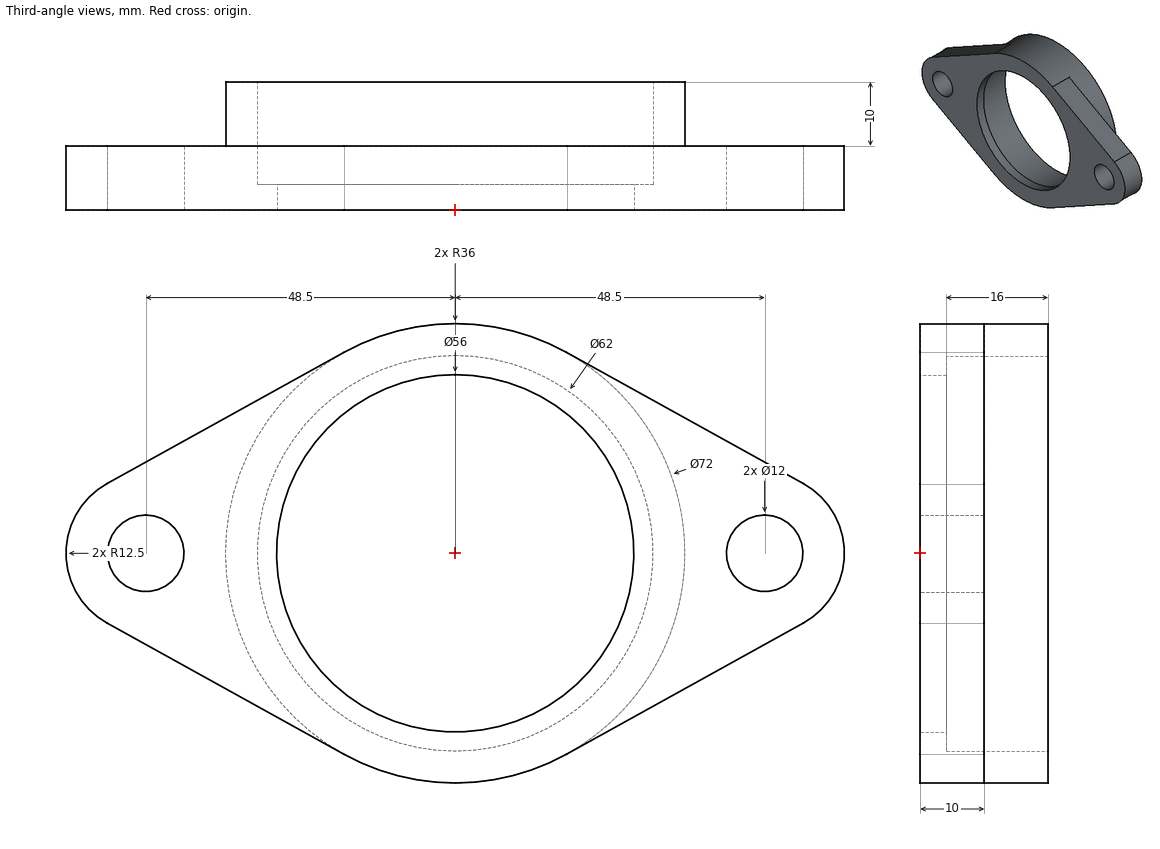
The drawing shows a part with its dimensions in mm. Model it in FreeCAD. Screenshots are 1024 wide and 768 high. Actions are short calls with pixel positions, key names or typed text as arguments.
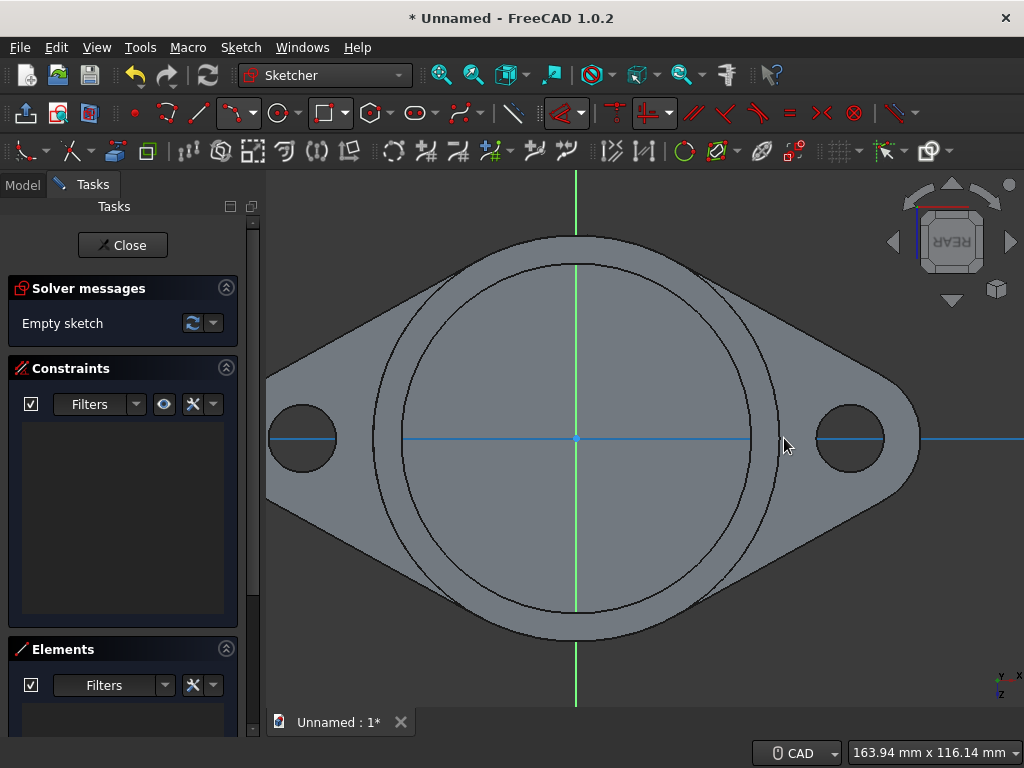
click(278, 114)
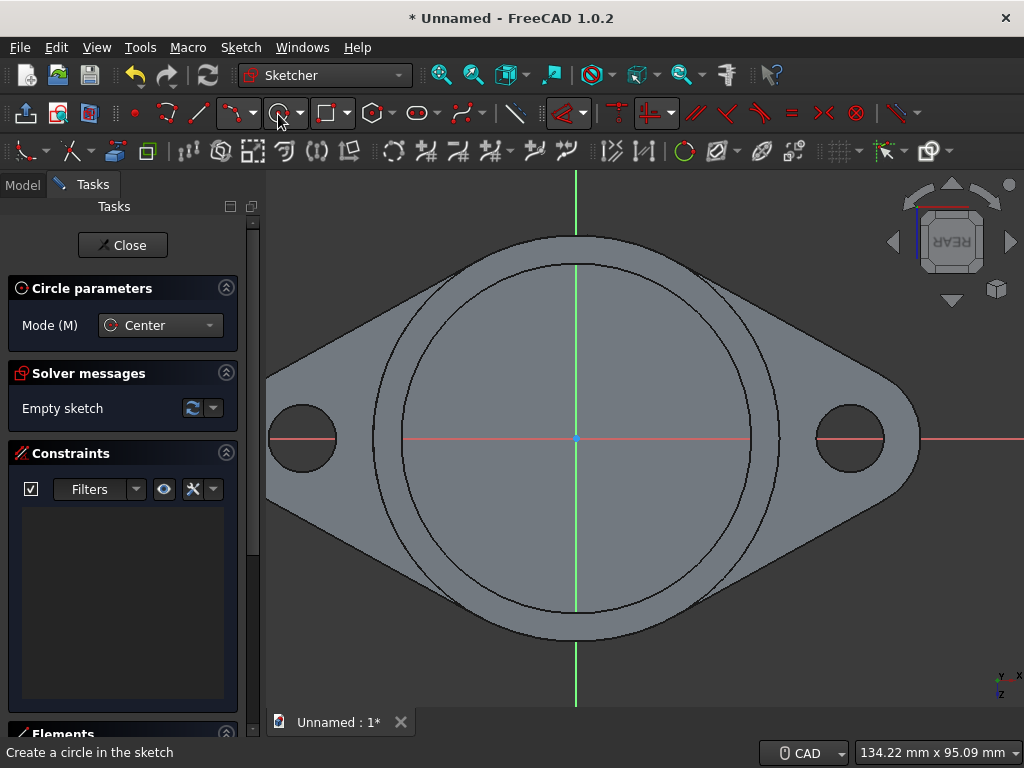
click(576, 438)
click(688, 327)
key(Escape)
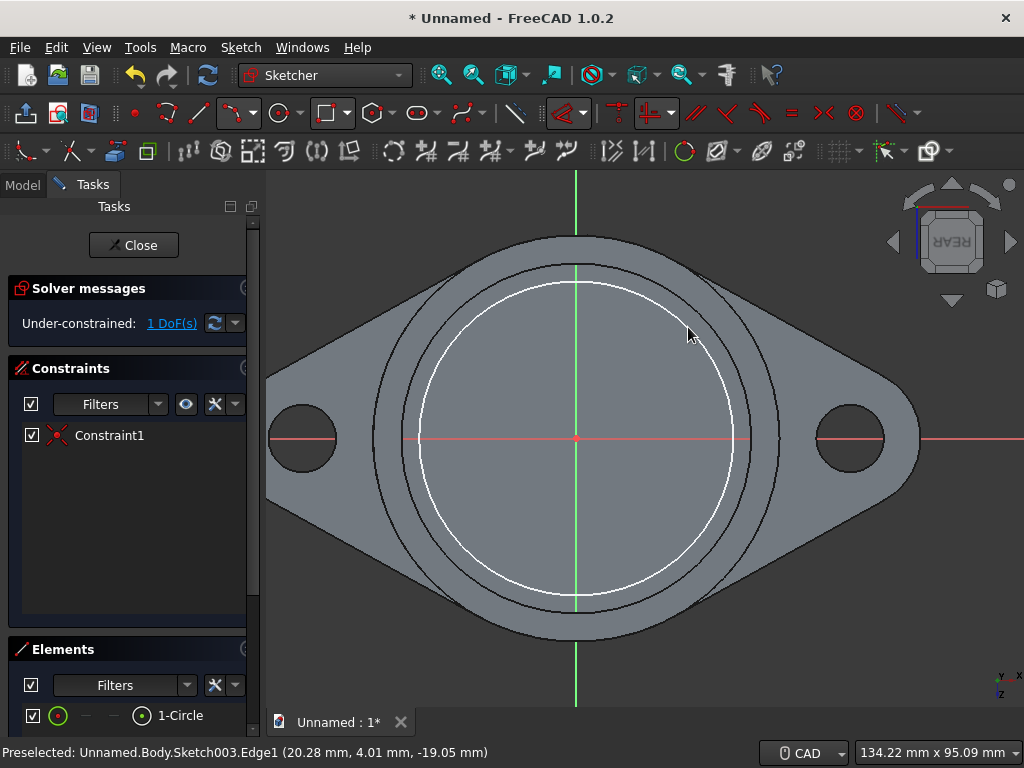
click(687, 327)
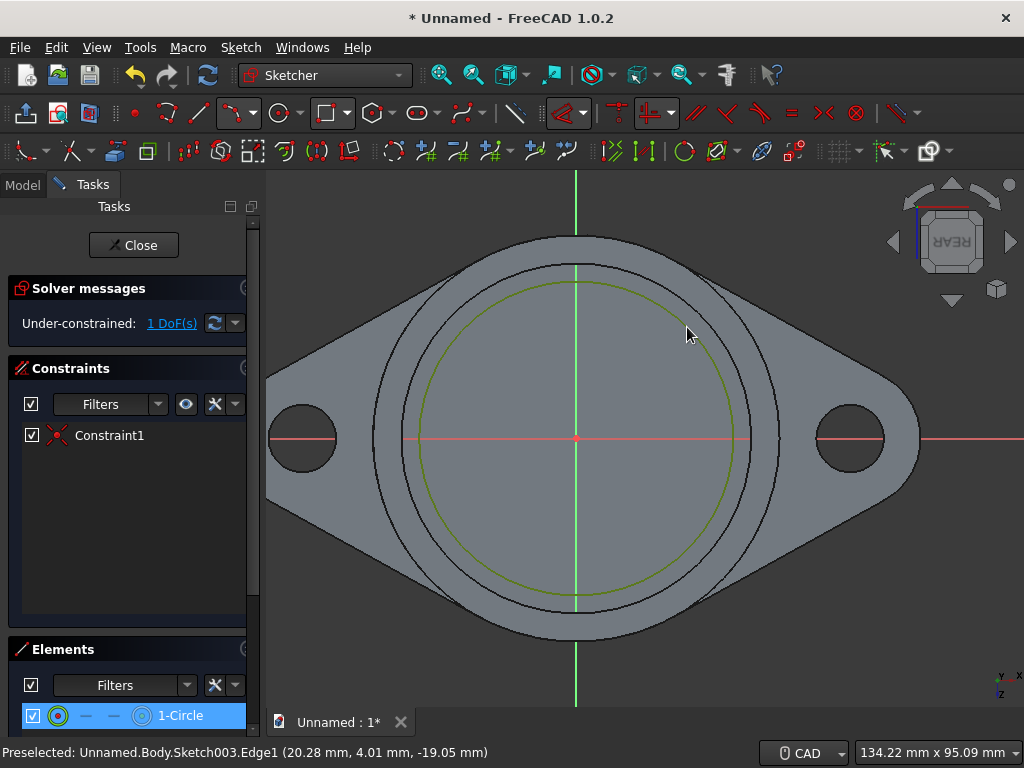
key(k)
key(o)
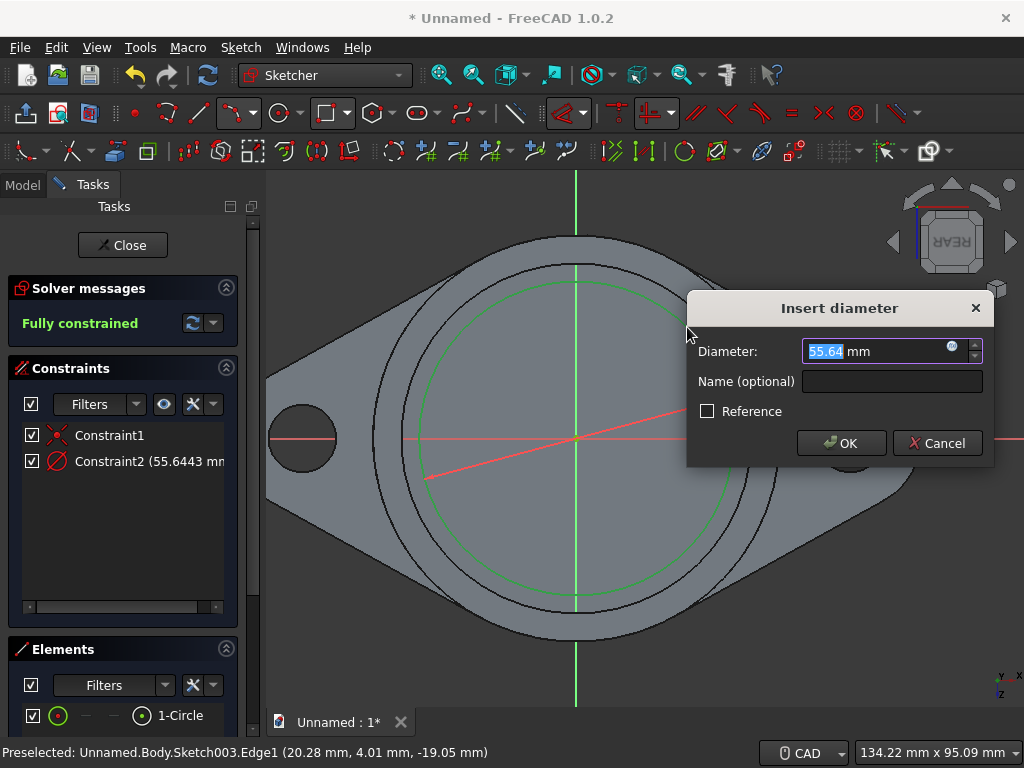
text(56)
key(Return)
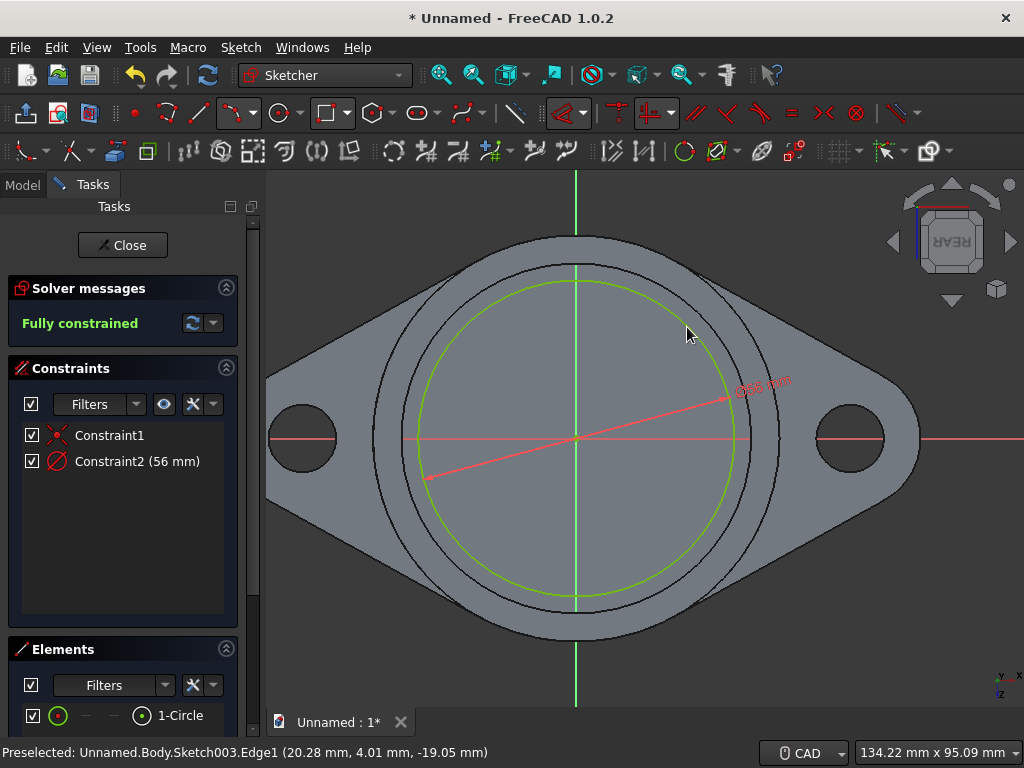
click(123, 245)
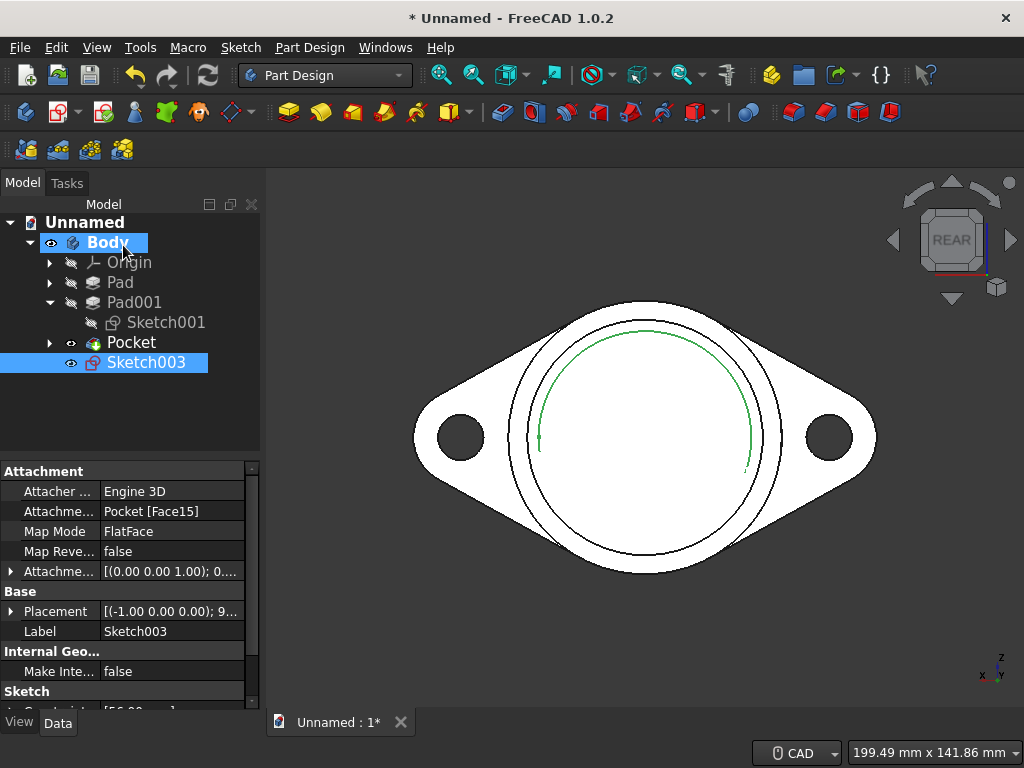
click(504, 112)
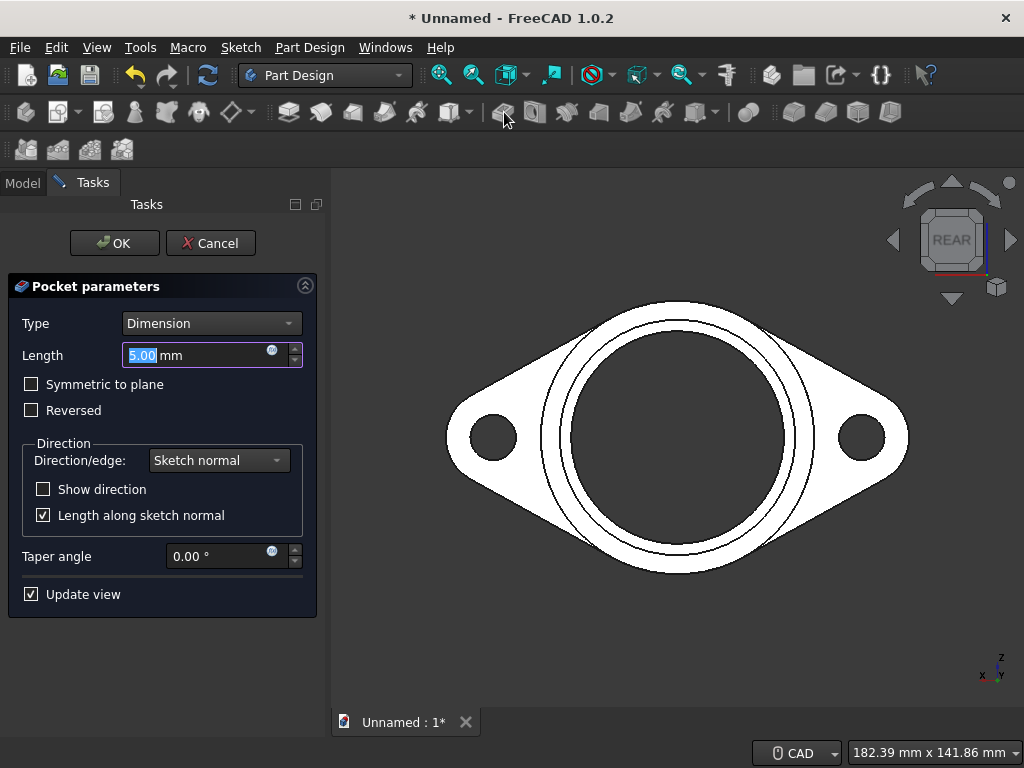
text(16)
key(Tab)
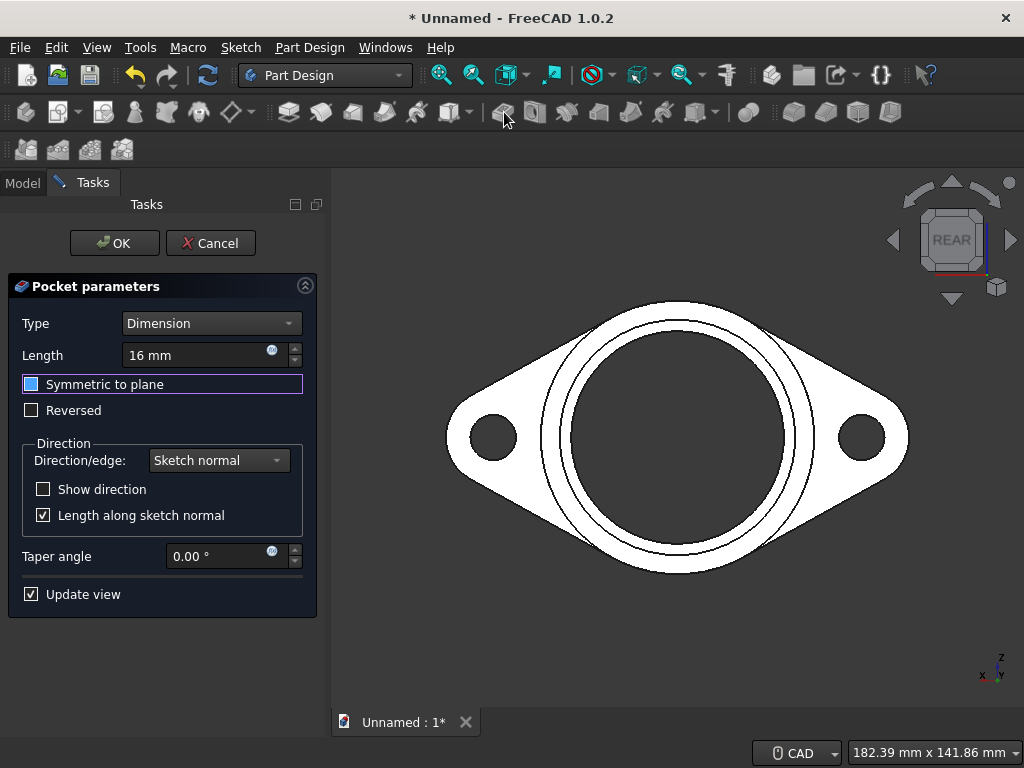
click(115, 243)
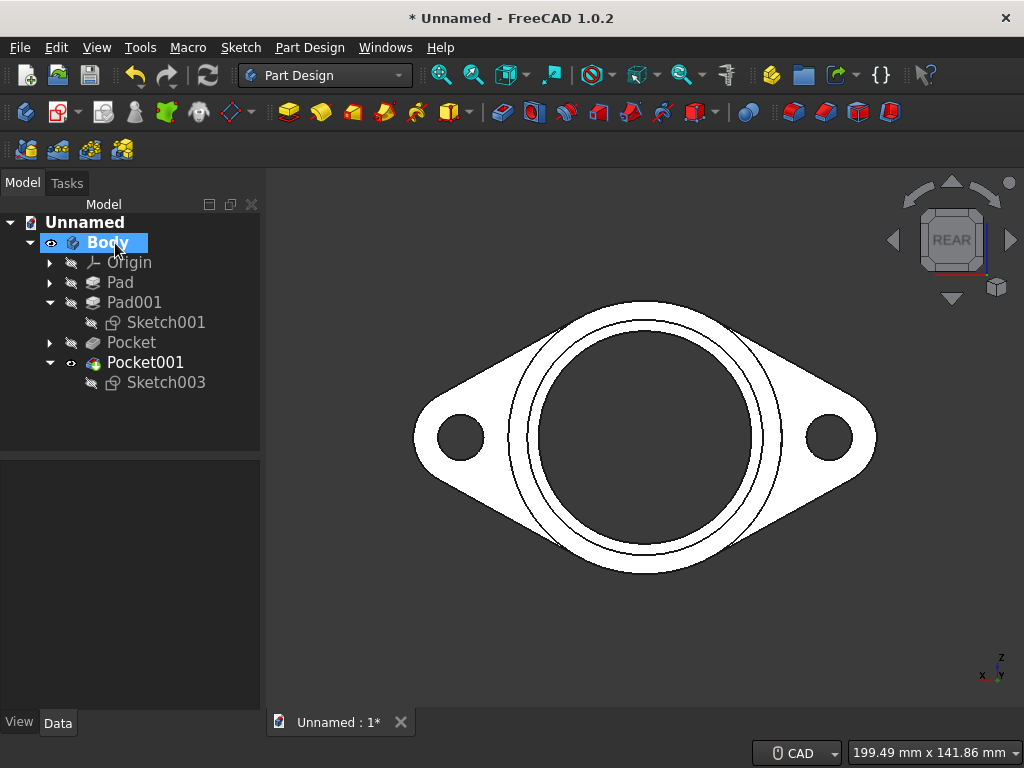
key(0)